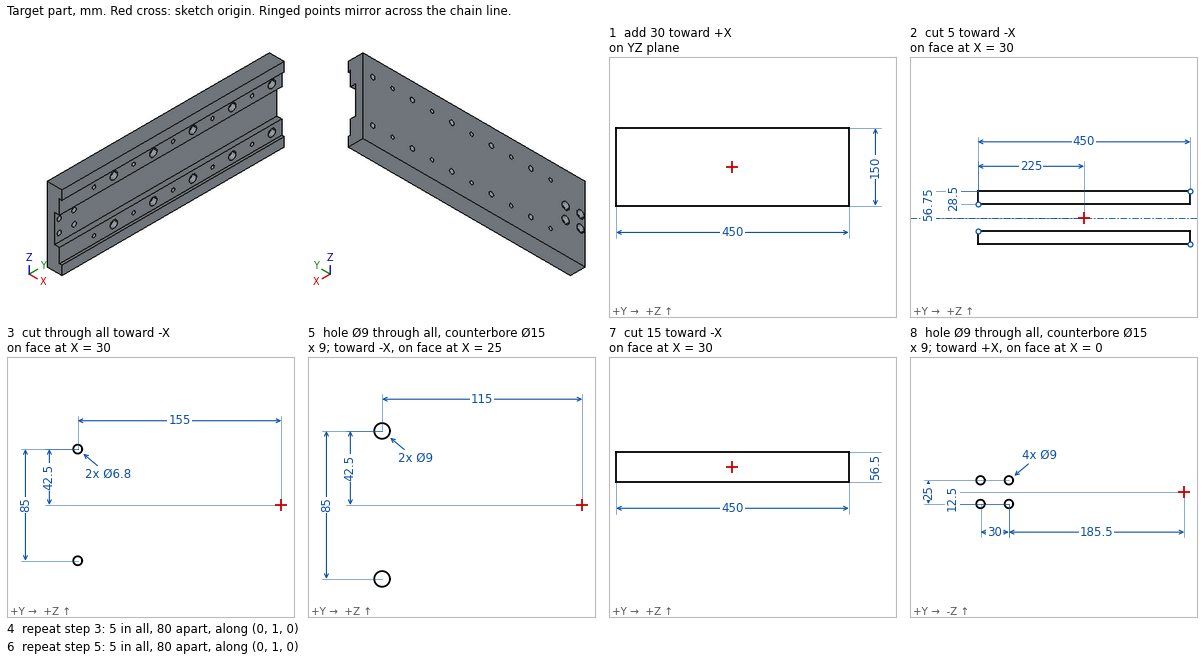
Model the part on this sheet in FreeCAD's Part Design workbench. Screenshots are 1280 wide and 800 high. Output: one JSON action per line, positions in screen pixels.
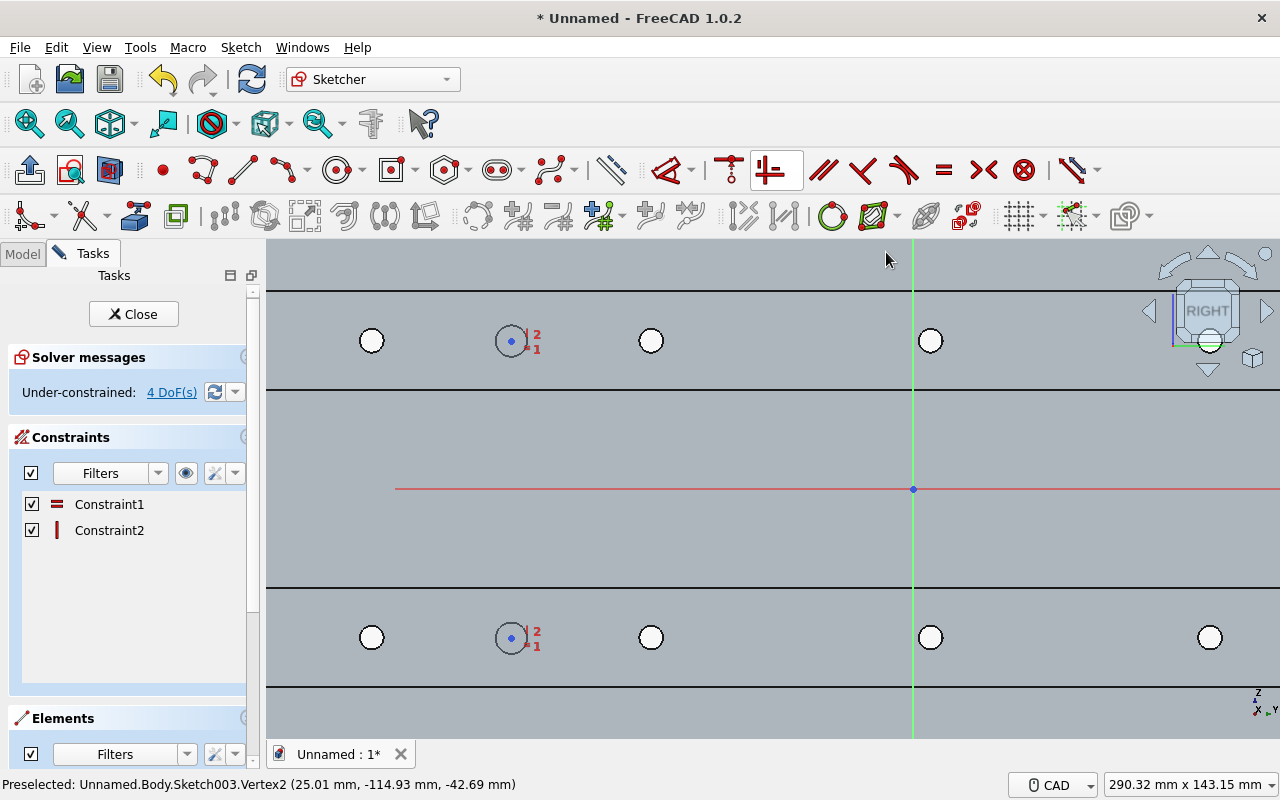
{"action": "left_click", "coordinate": [666, 170]}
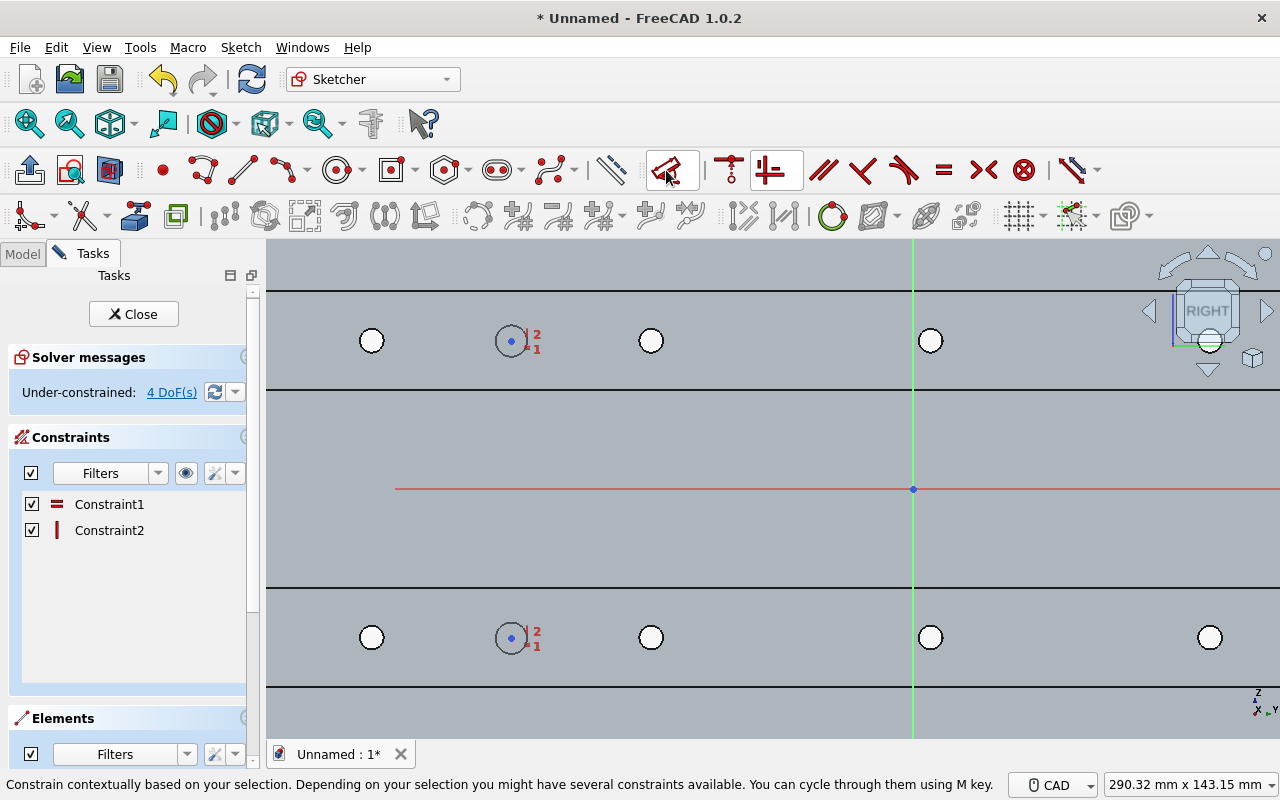
{"action": "scroll", "coordinate": [522, 330], "scroll_direction": "up", "scroll_amount": 2}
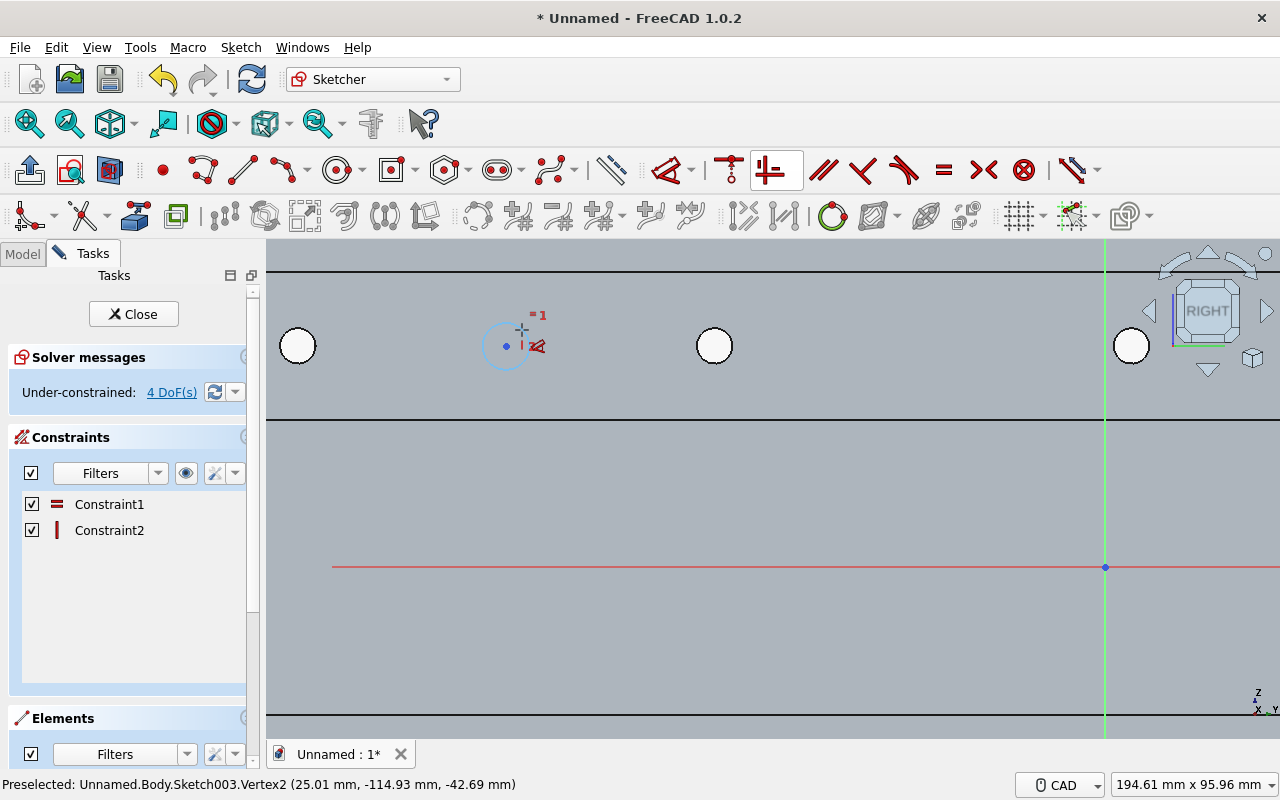
{"action": "left_click", "coordinate": [523, 330]}
{"action": "left_click", "coordinate": [546, 308]}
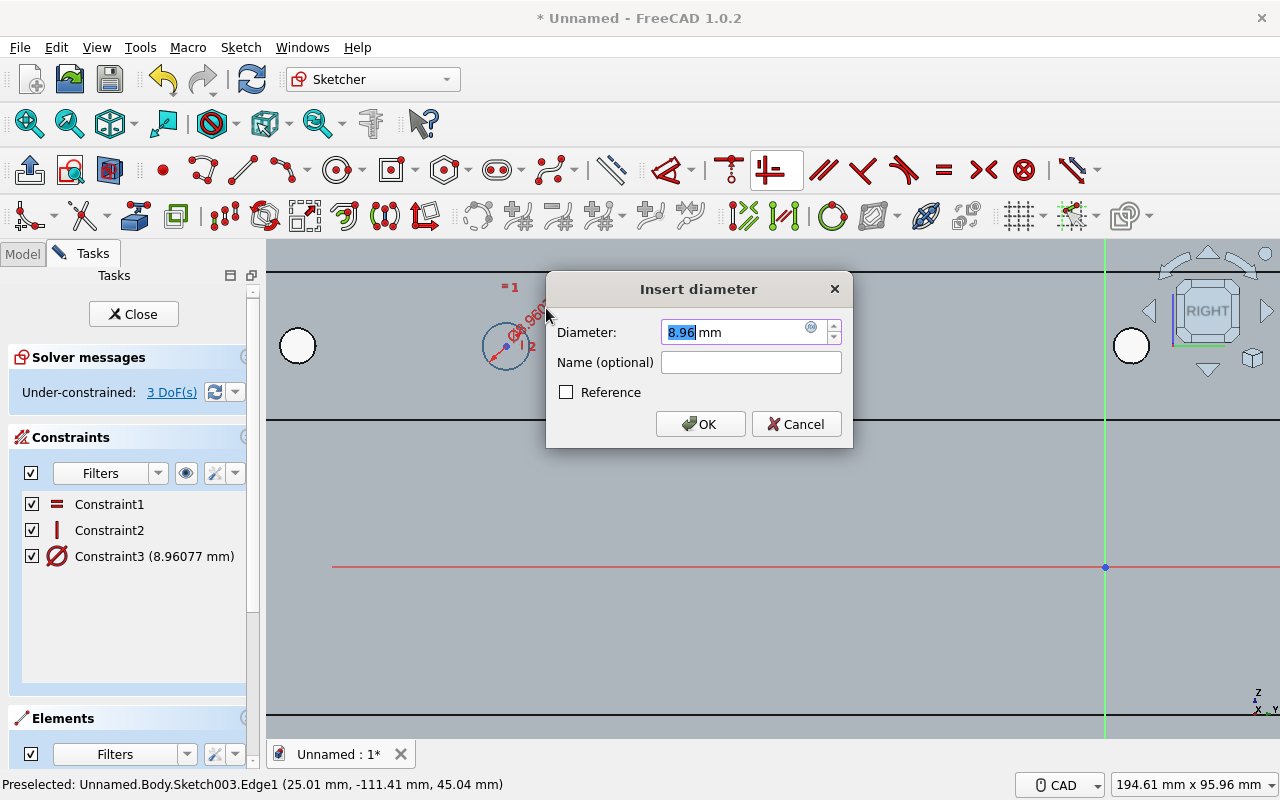
{"action": "type", "text": "9"}
{"action": "key", "text": "Return"}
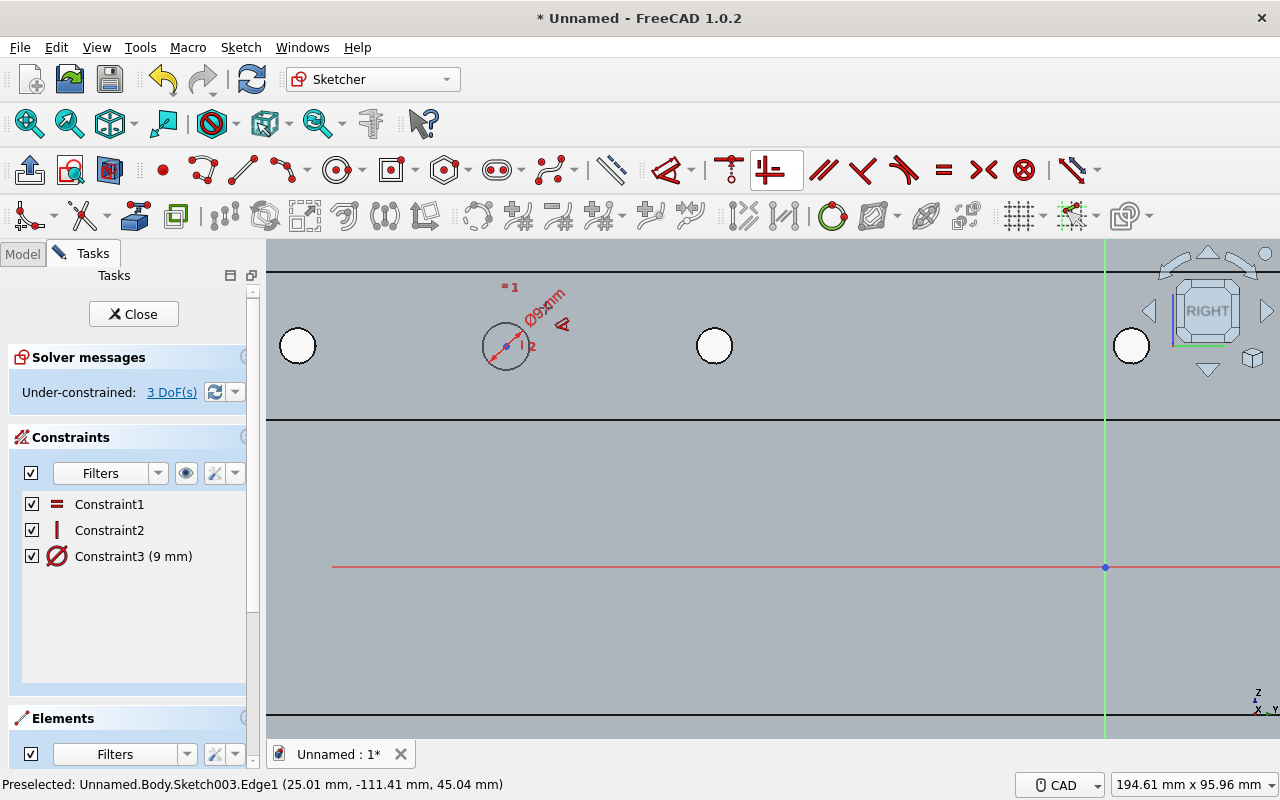
{"action": "left_click", "coordinate": [506, 346]}
{"action": "left_click", "coordinate": [806, 312]}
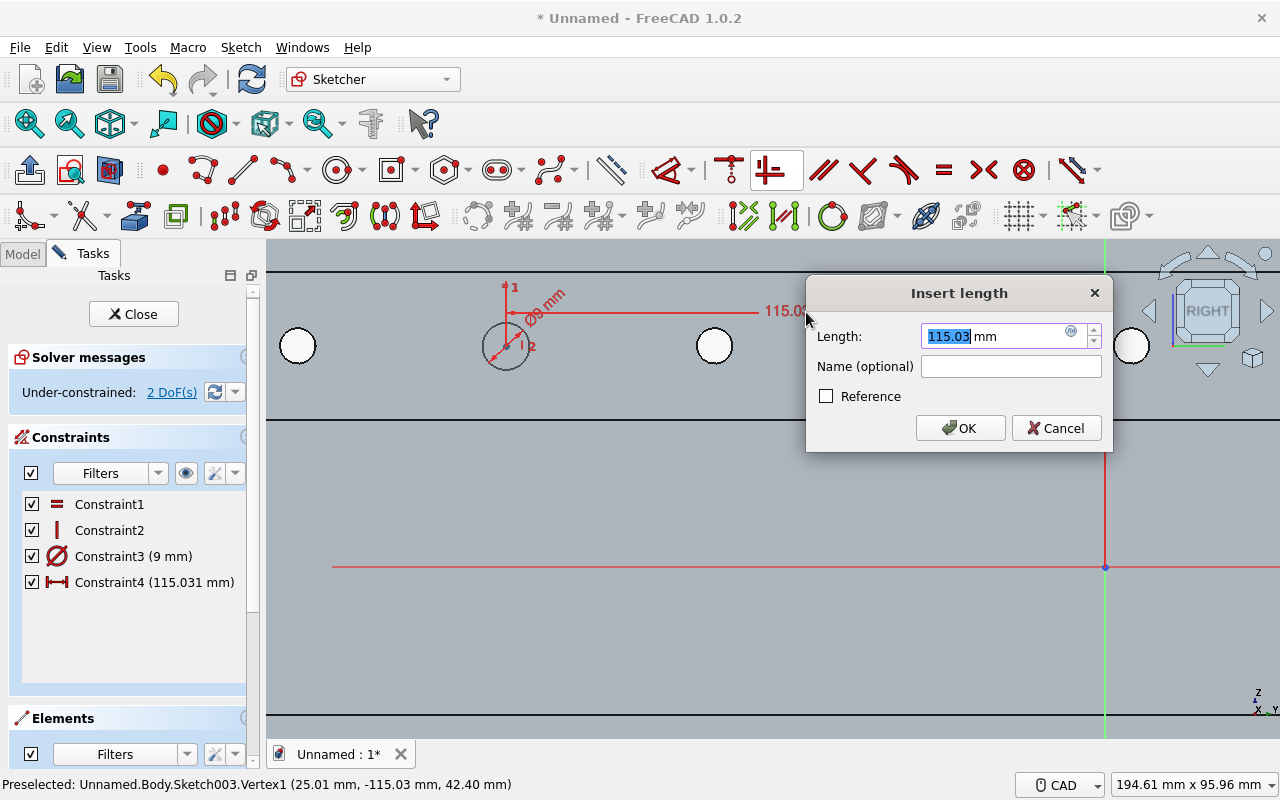
{"action": "type", "text": "115"}
{"action": "key", "text": "Return"}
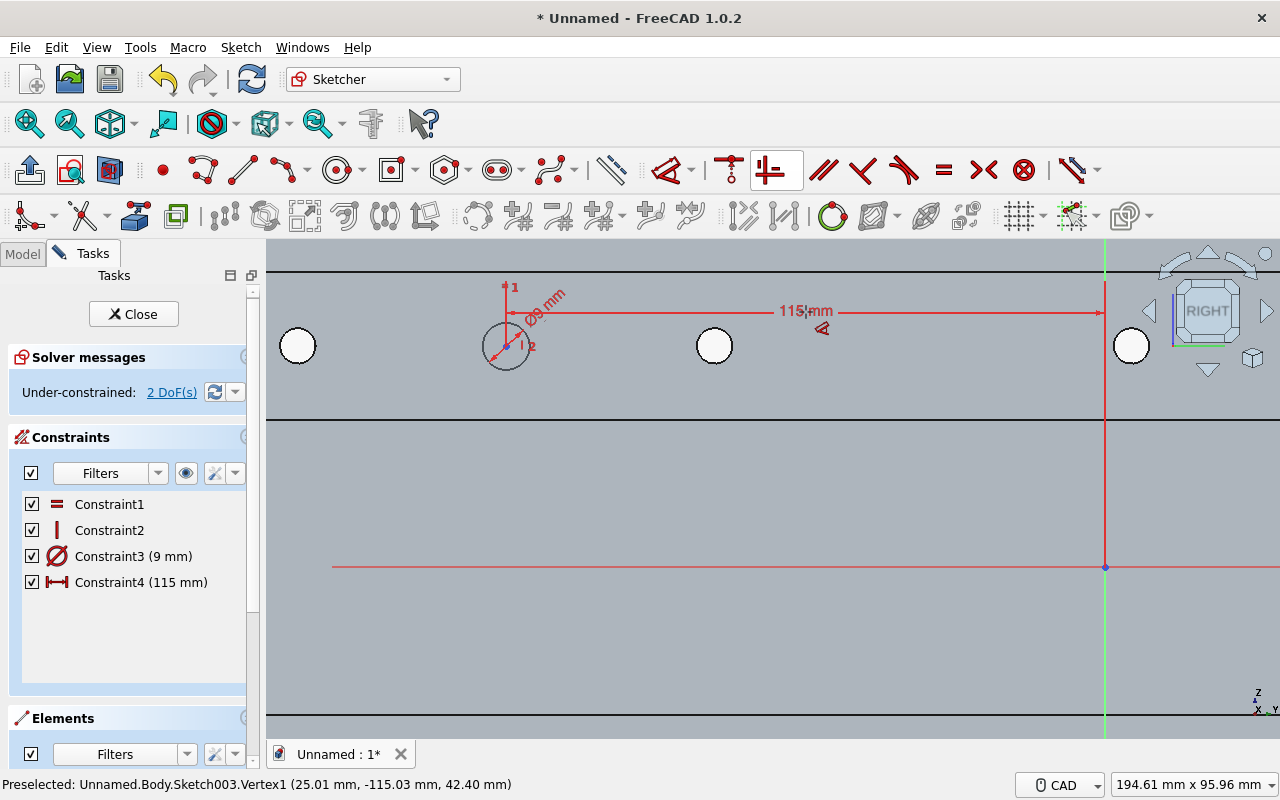
{"action": "left_click", "coordinate": [506, 346]}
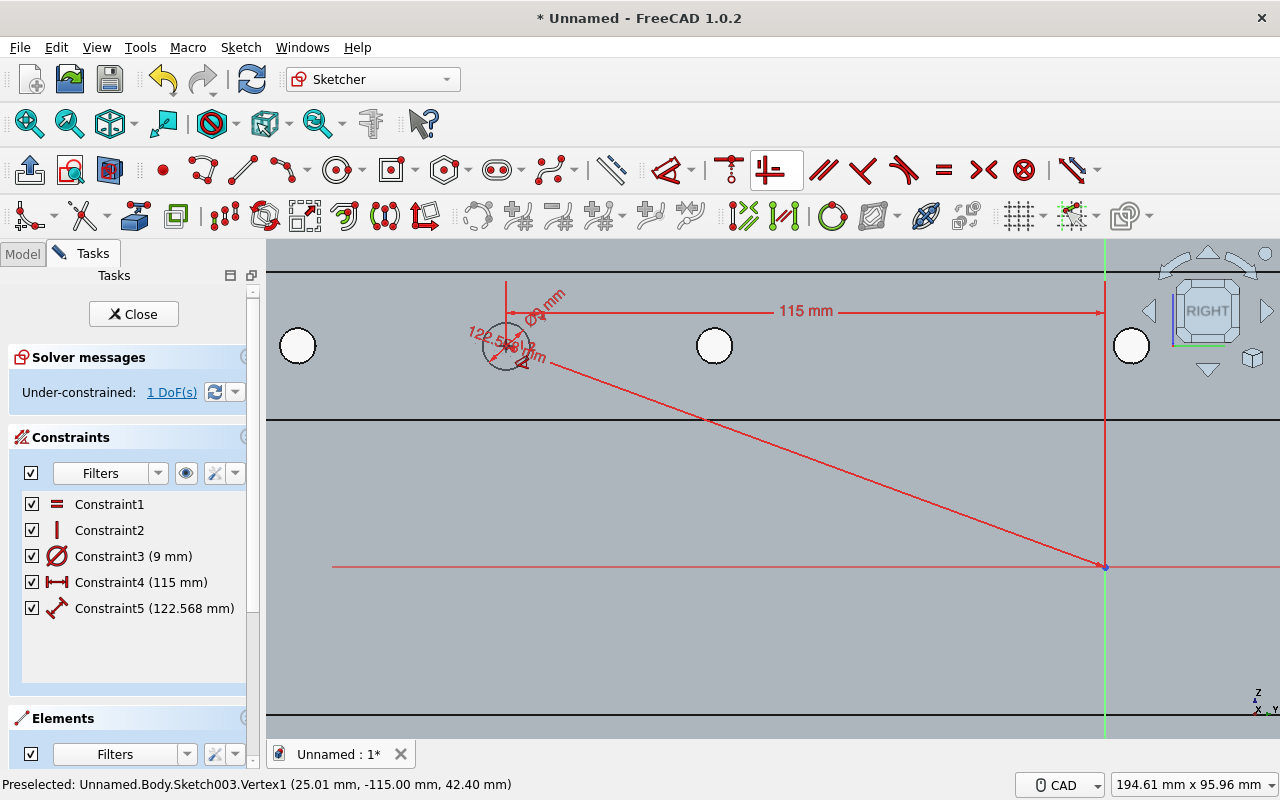
{"action": "scroll", "coordinate": [522, 330], "scroll_direction": "down", "scroll_amount": 2}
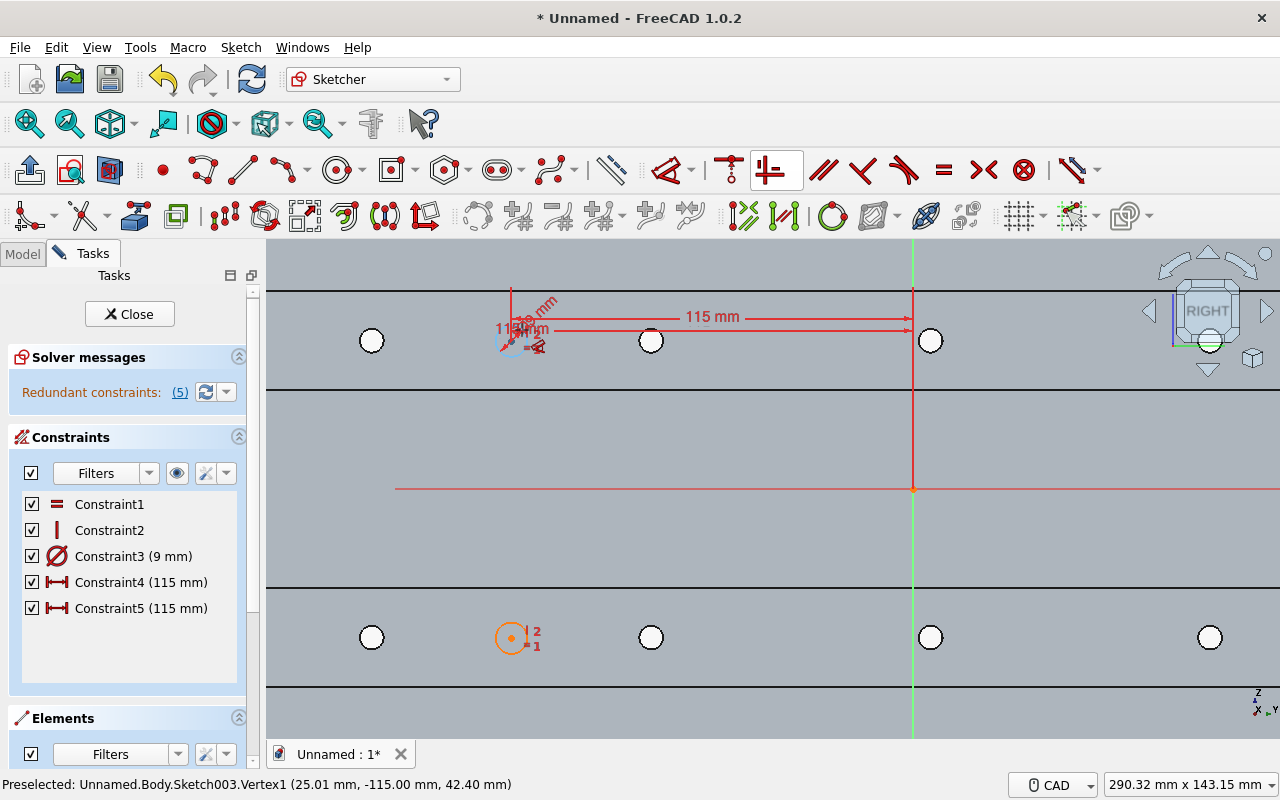
{"action": "left_click", "coordinate": [511, 638]}
{"action": "left_click", "coordinate": [477, 421]}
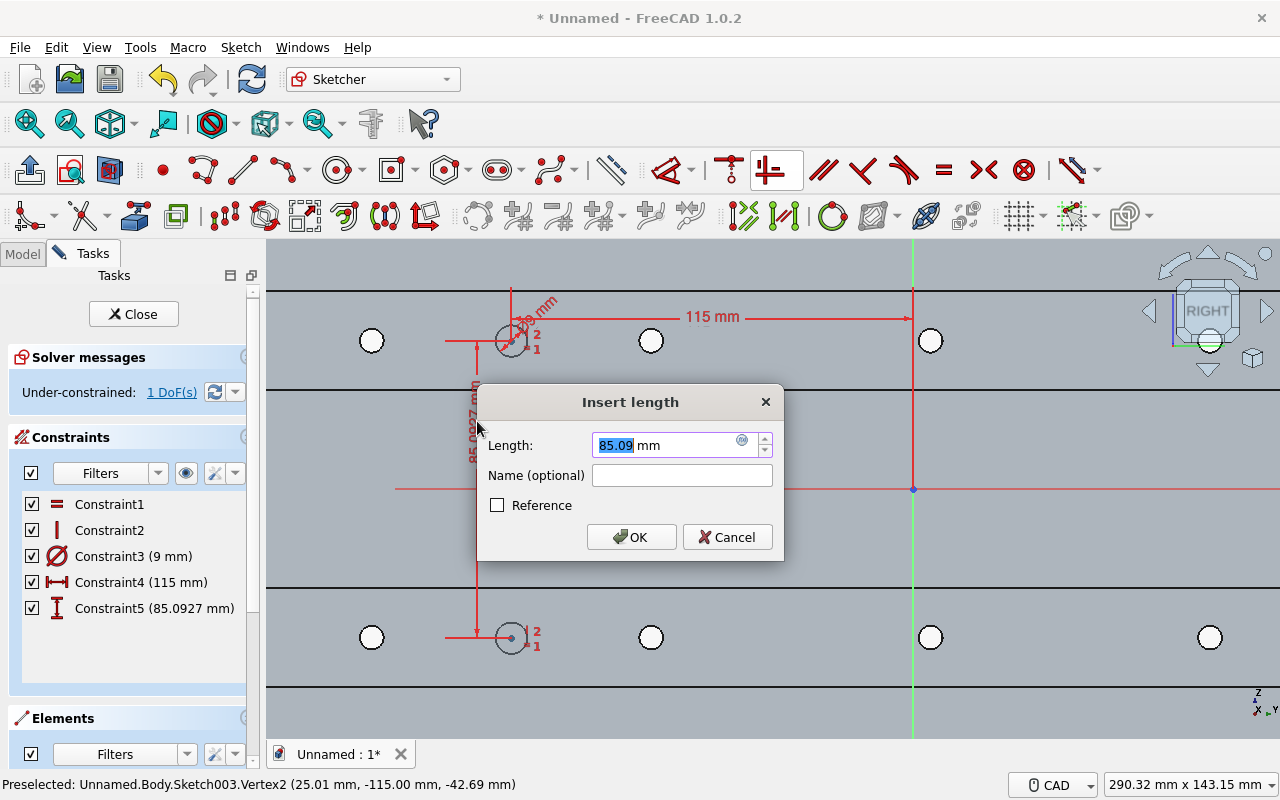
{"action": "type", "text": "85"}
{"action": "key", "text": "Return"}